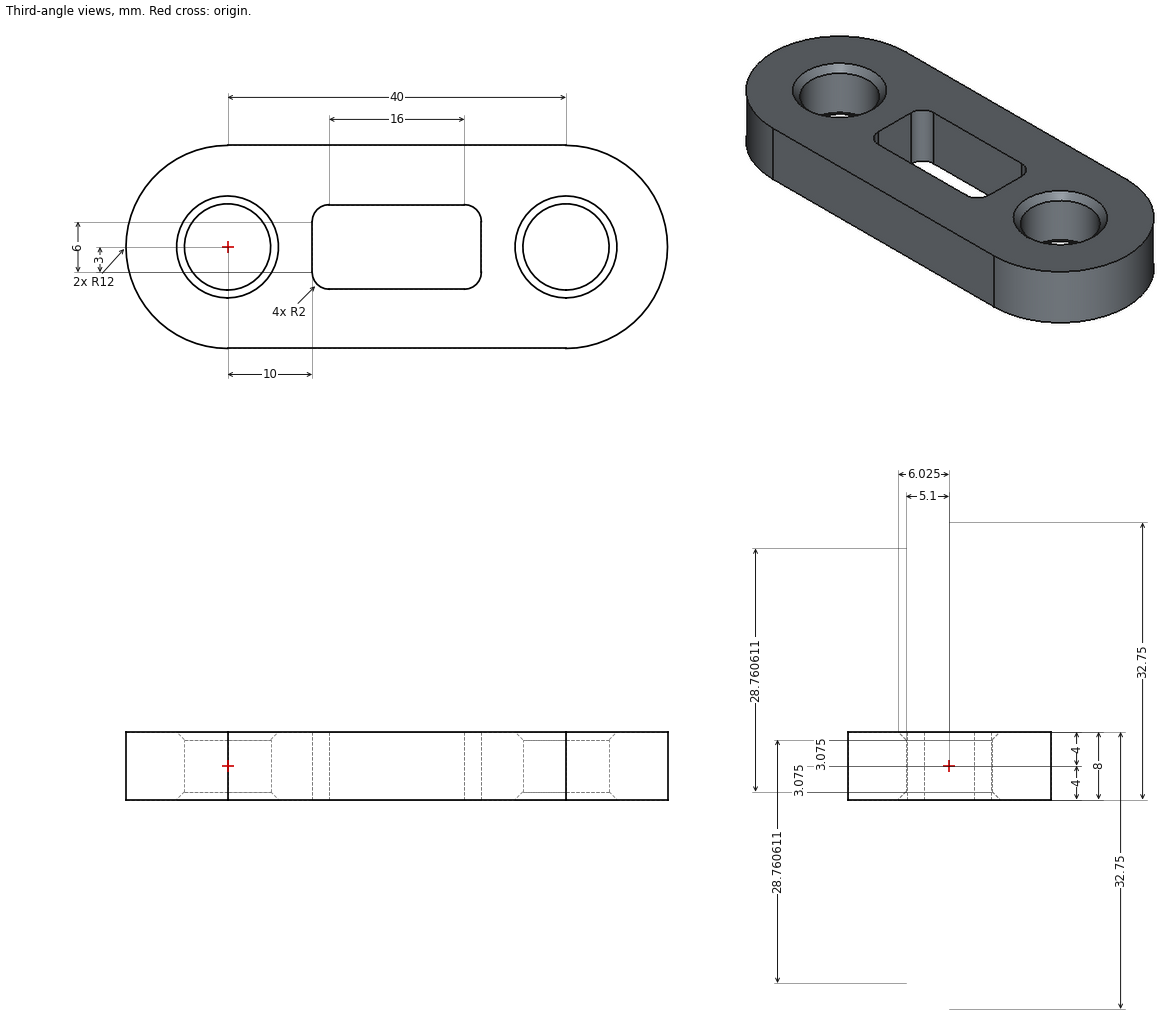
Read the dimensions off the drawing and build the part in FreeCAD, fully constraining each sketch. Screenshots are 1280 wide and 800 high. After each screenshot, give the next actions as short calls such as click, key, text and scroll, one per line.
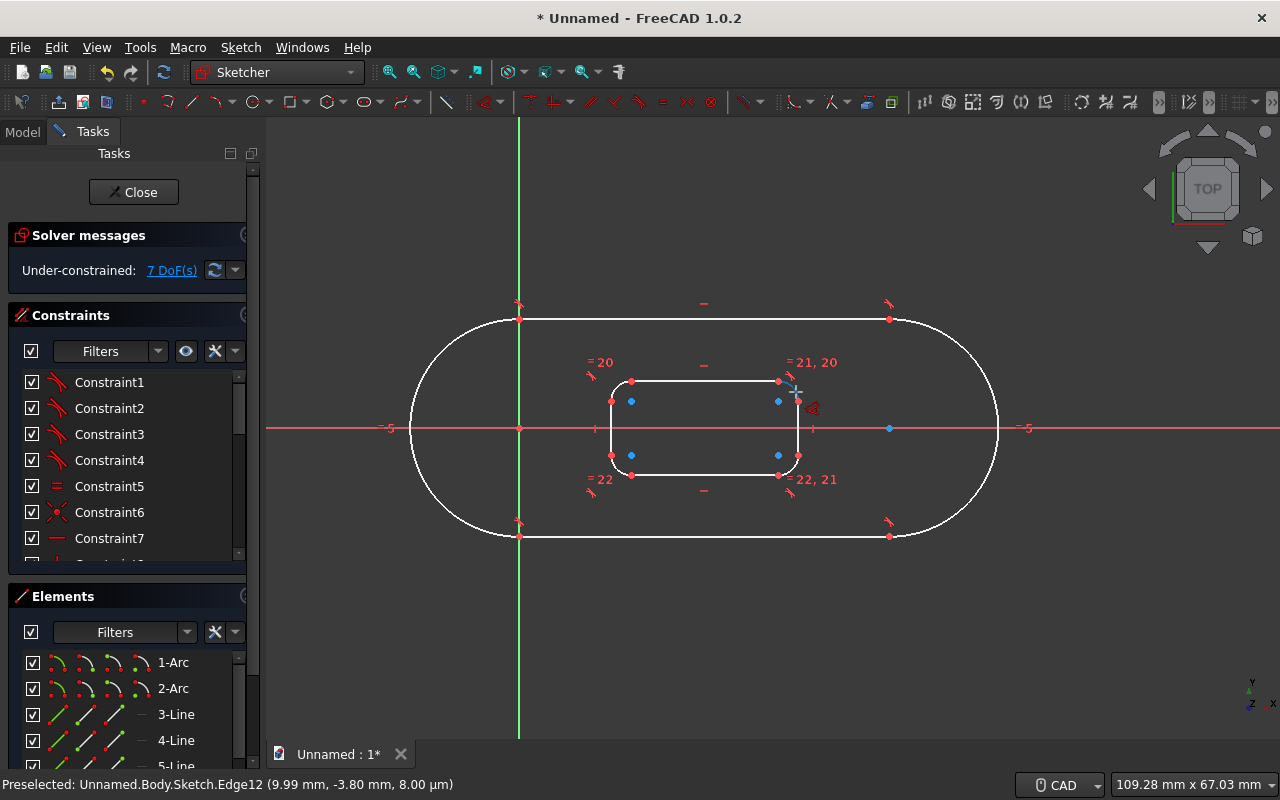
click(431, 364)
click(405, 345)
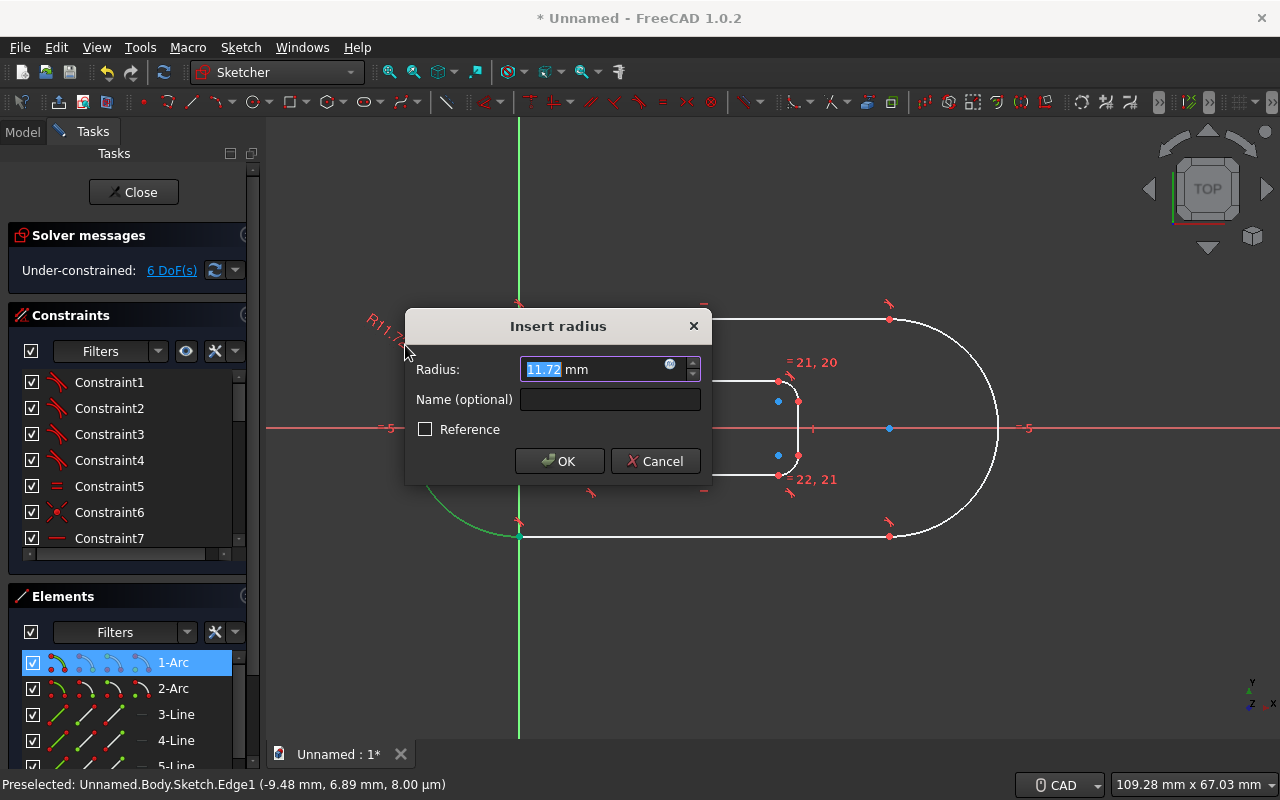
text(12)
key(Return)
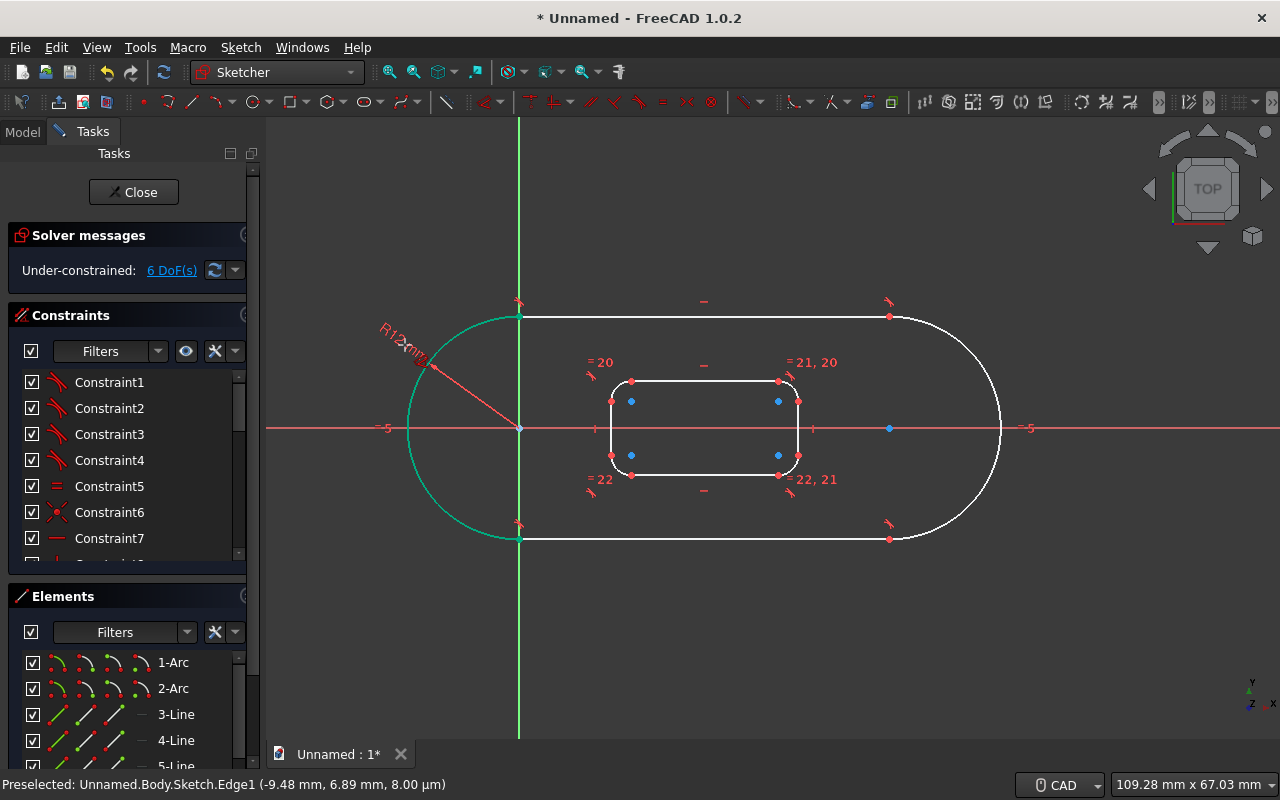
scroll(622, 383, up, 4)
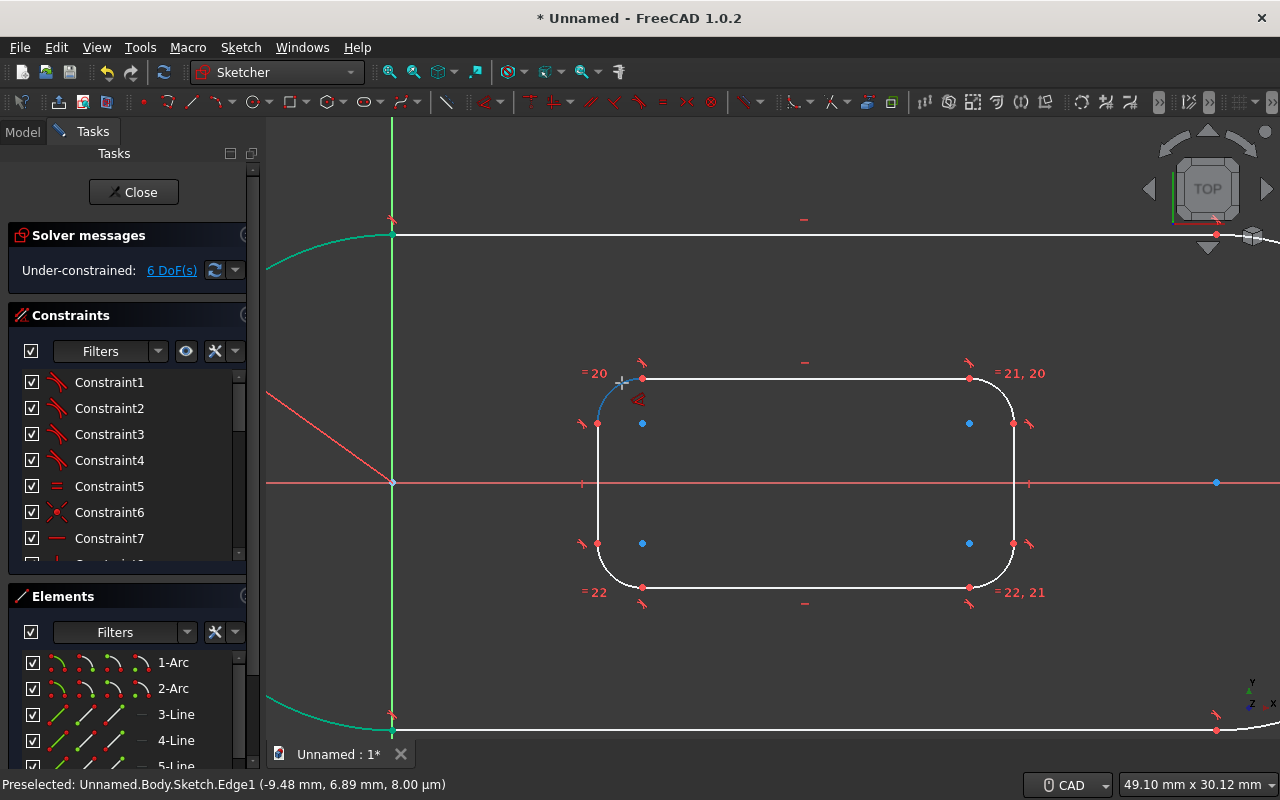
click(622, 383)
click(608, 354)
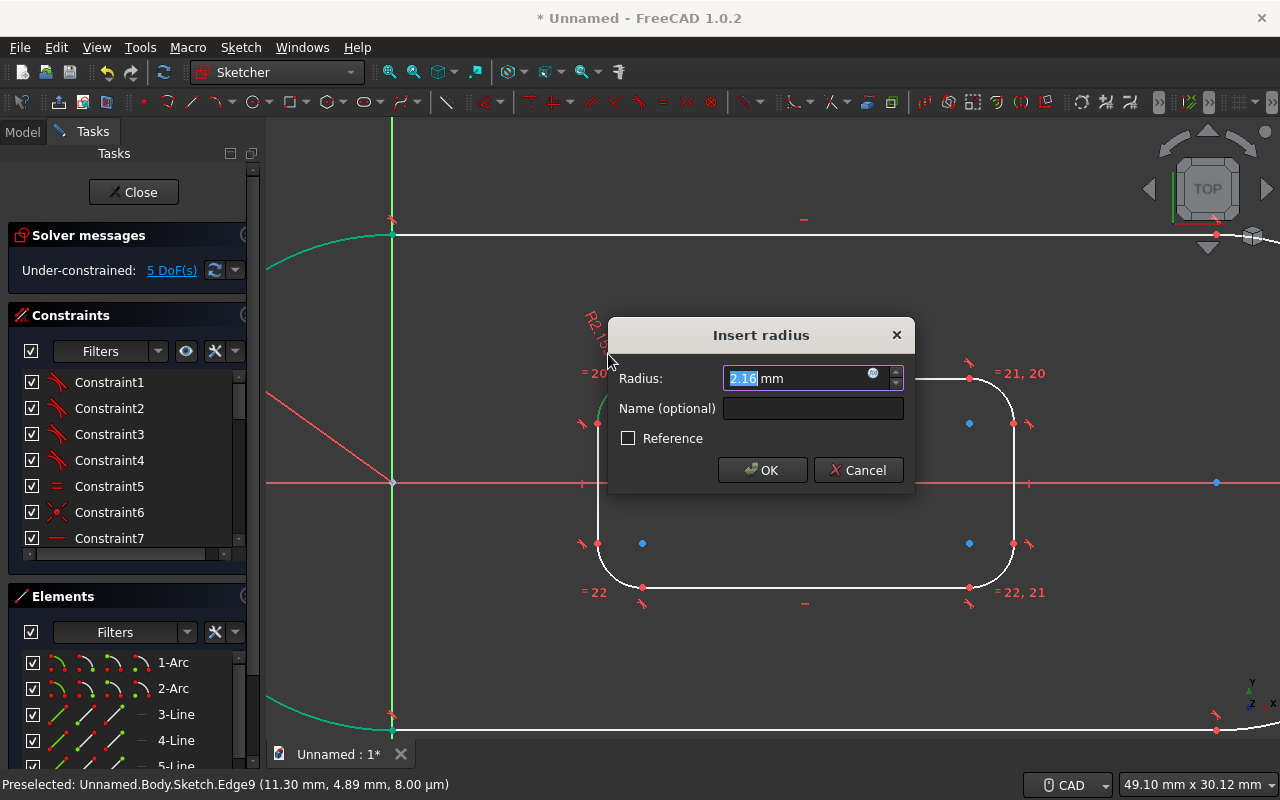
text(2)
key(Return)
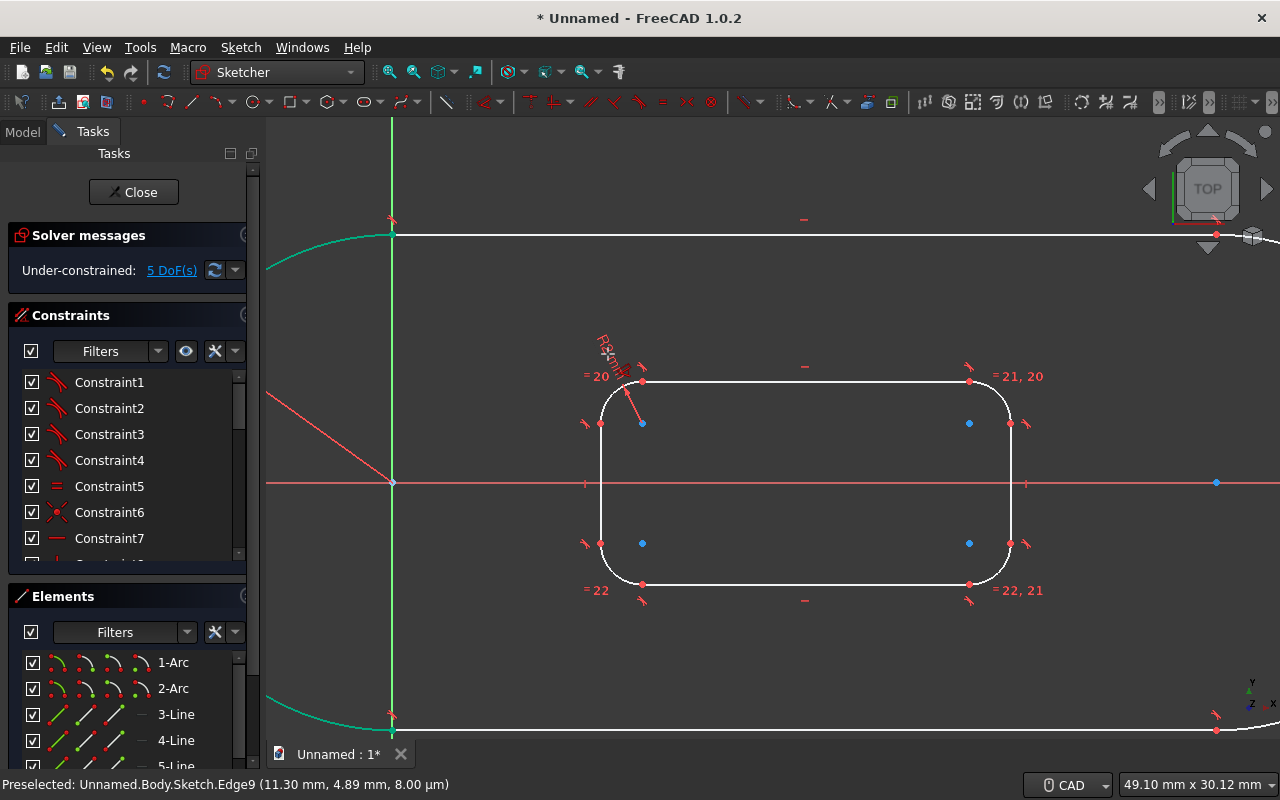
click(601, 507)
click(567, 455)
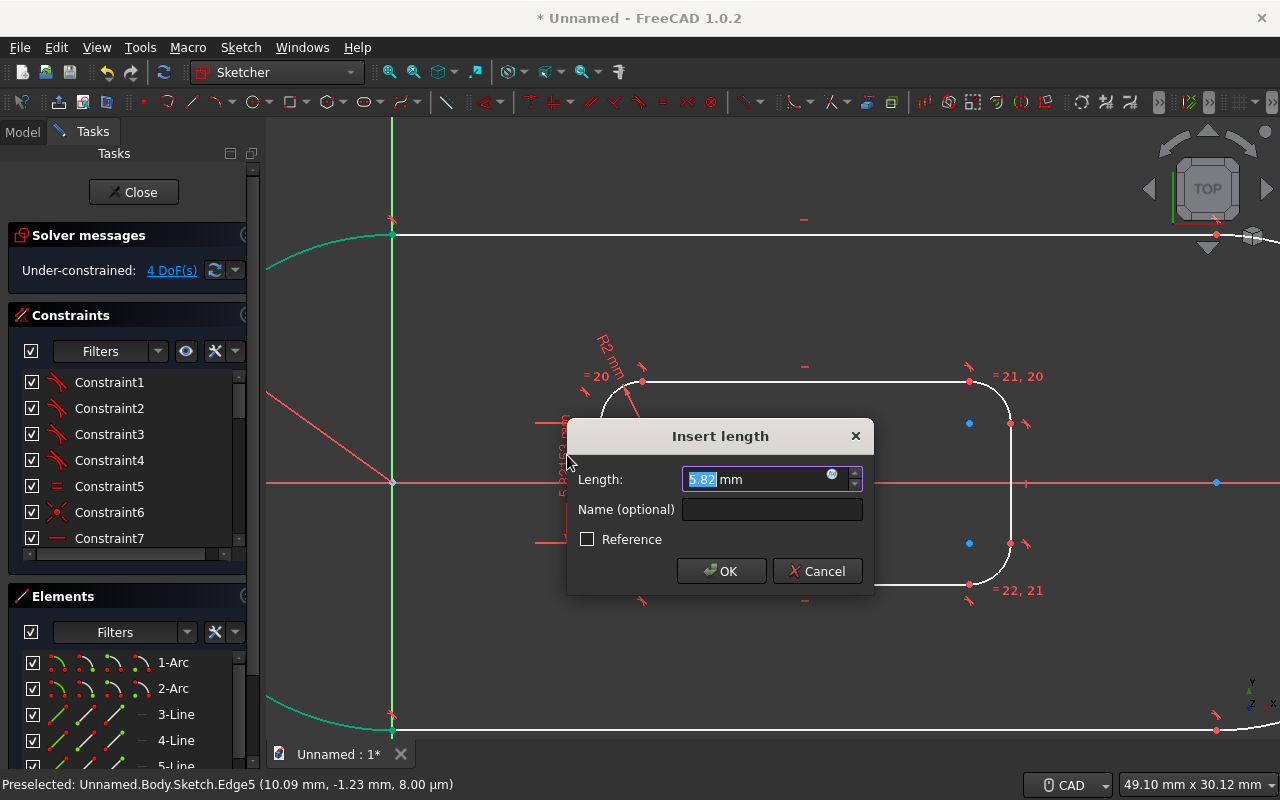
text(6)
key(Return)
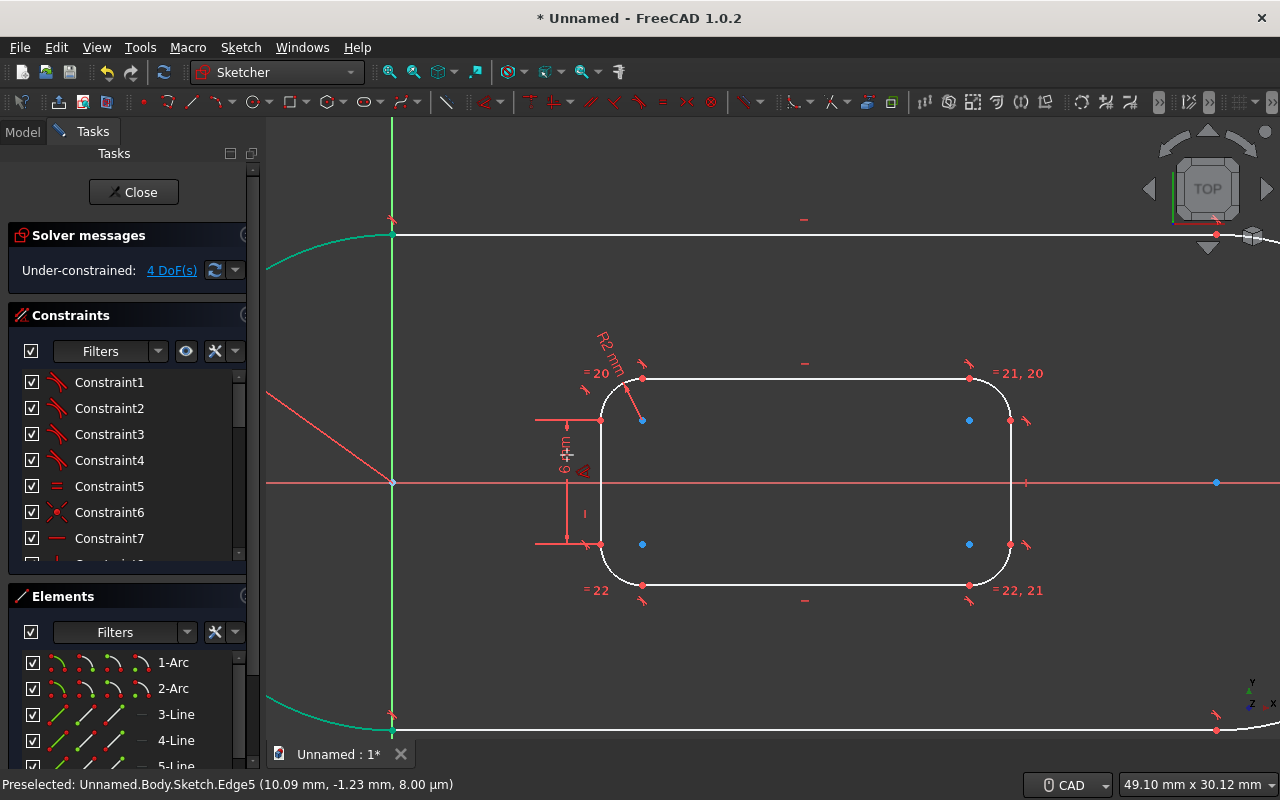
click(640, 235)
click(754, 201)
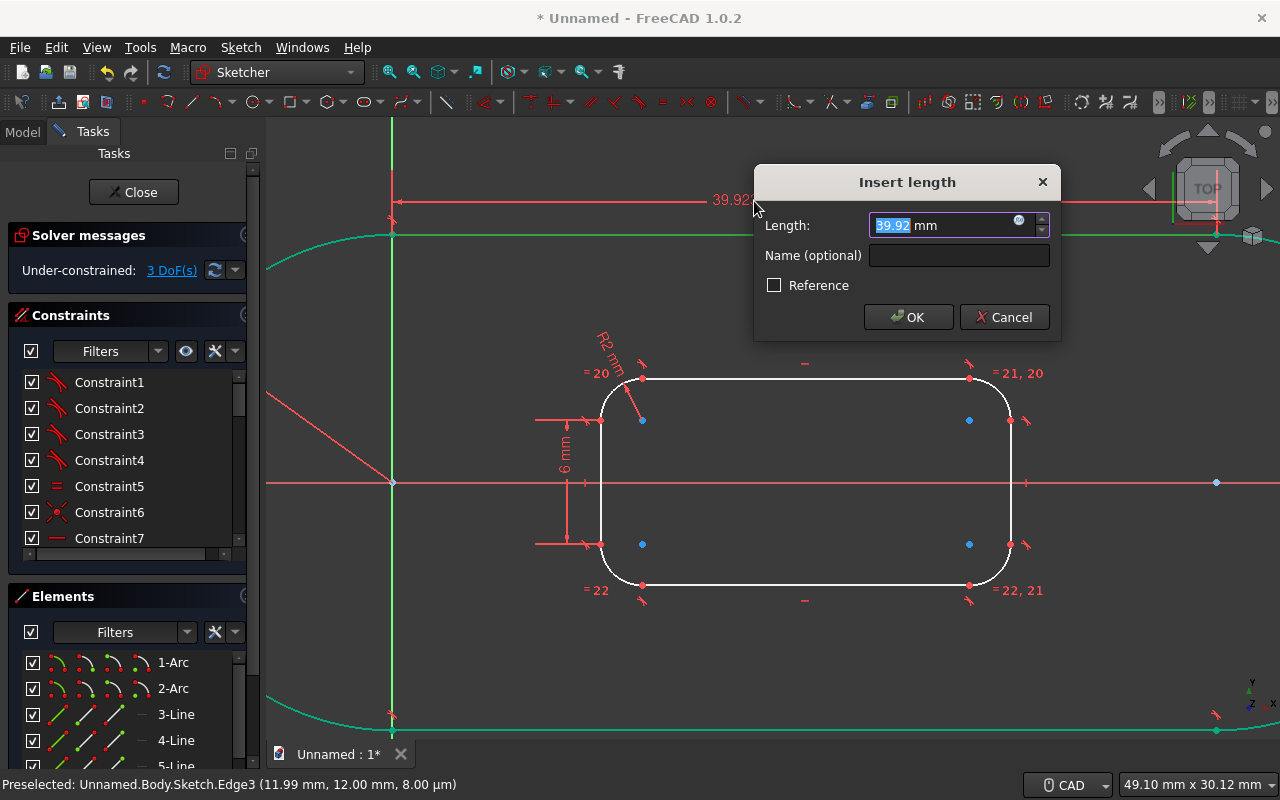
text(40)
key(Return)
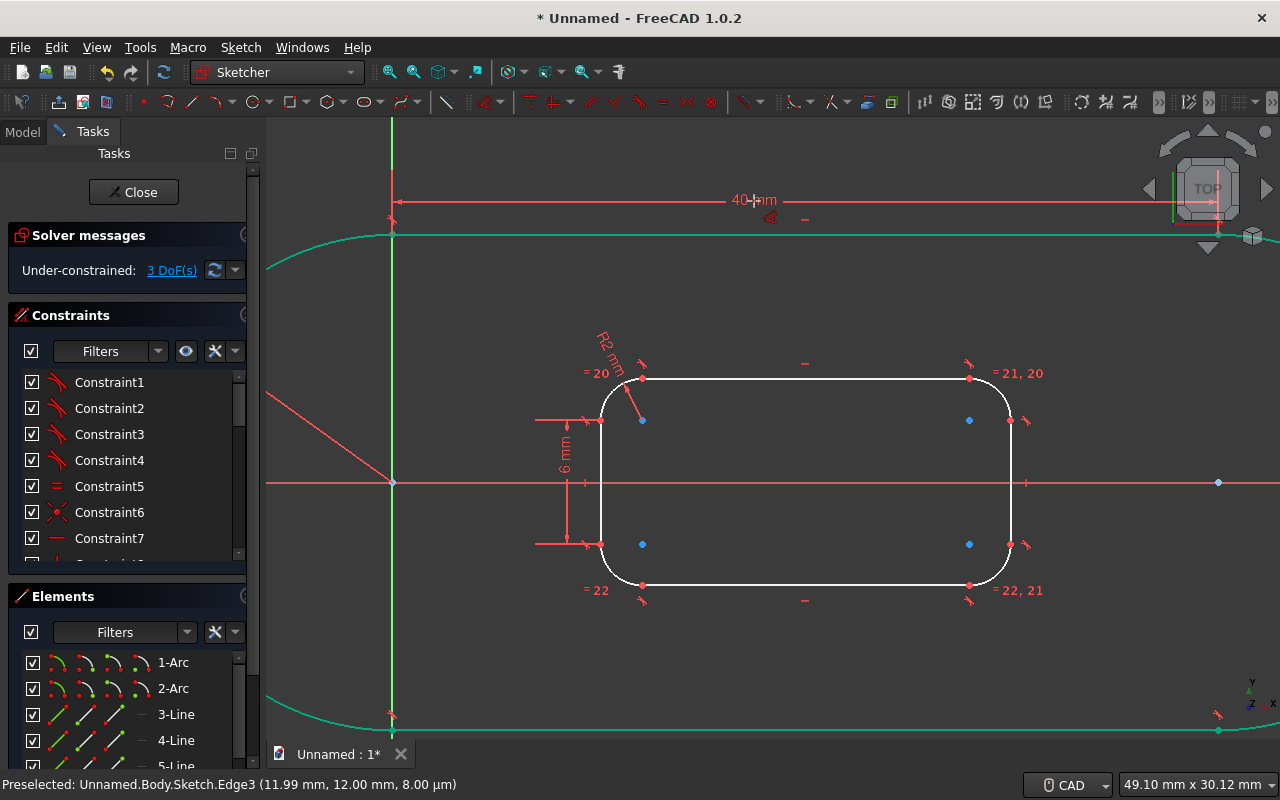
click(740, 379)
click(806, 345)